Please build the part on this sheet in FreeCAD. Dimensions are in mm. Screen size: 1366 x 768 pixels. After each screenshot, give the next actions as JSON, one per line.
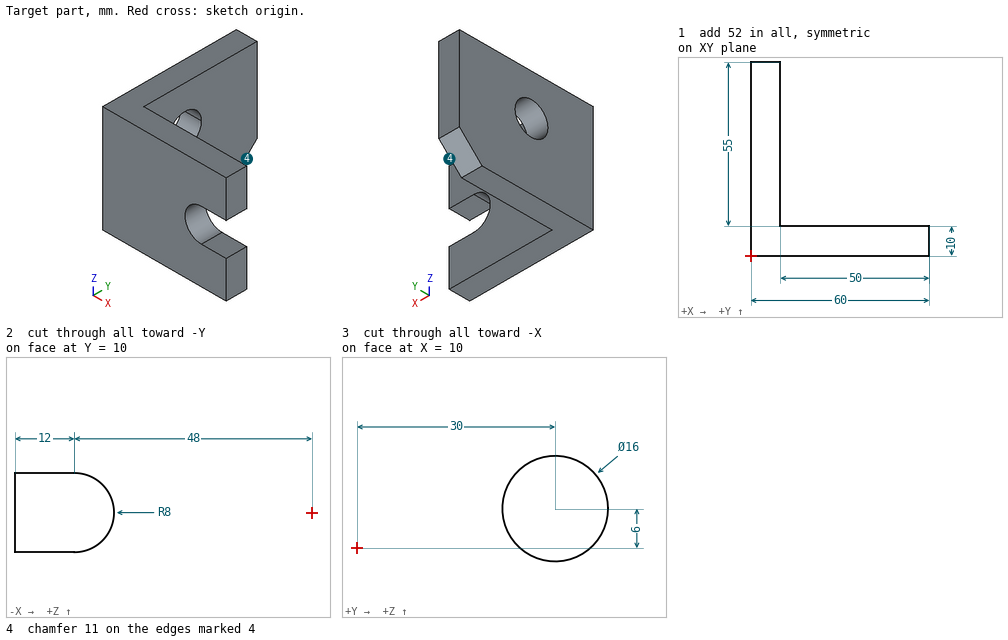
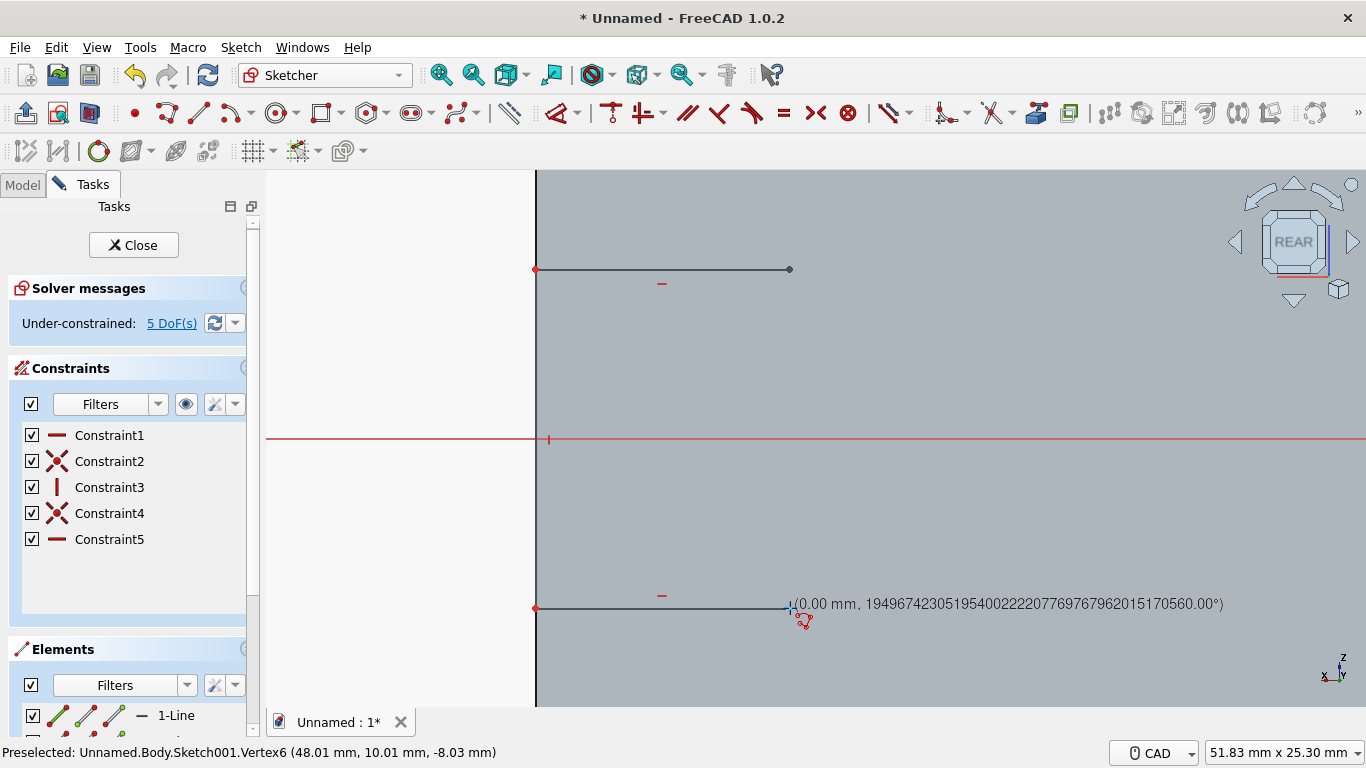
{"action": "key", "text": "g 3 a"}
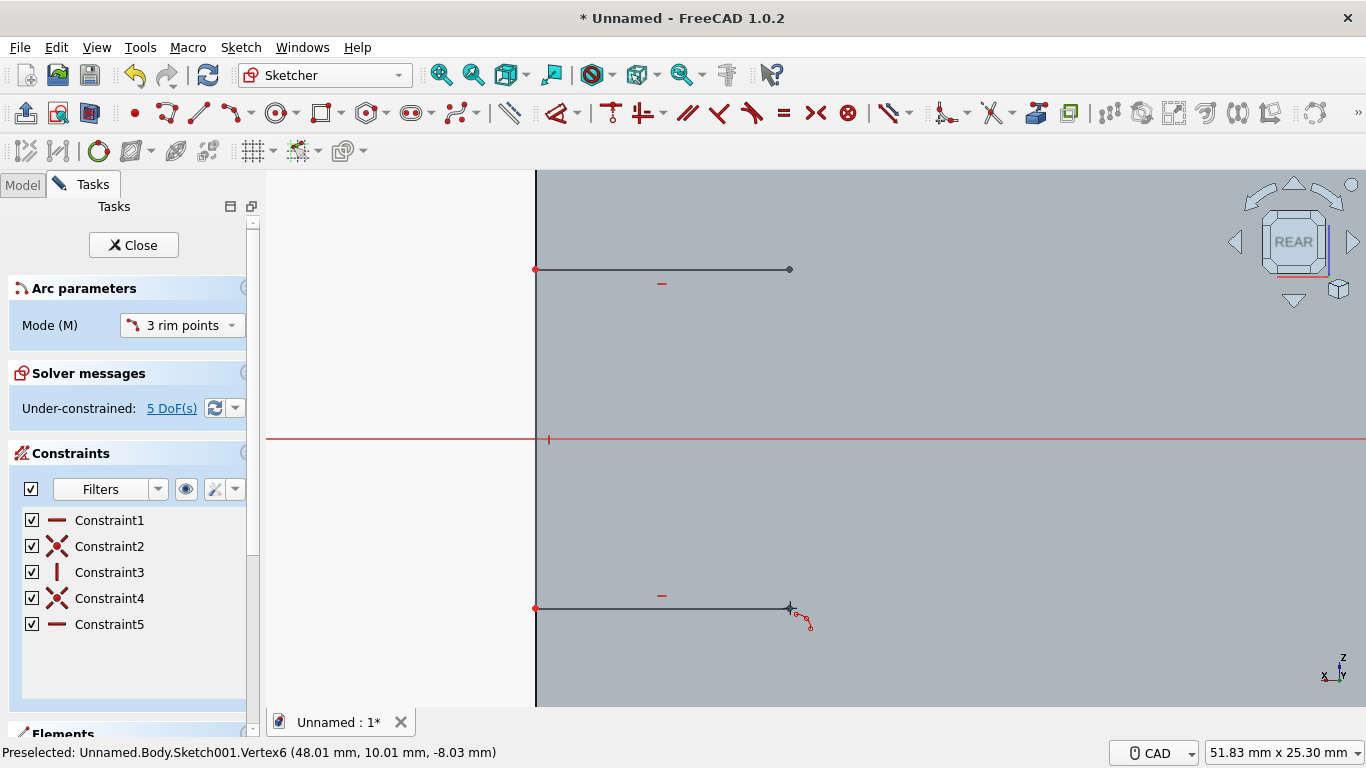
{"action": "left_click", "coordinate": [790, 609]}
{"action": "left_click", "coordinate": [790, 270]}
{"action": "left_click", "coordinate": [952, 491]}
{"action": "key", "text": "Escape"}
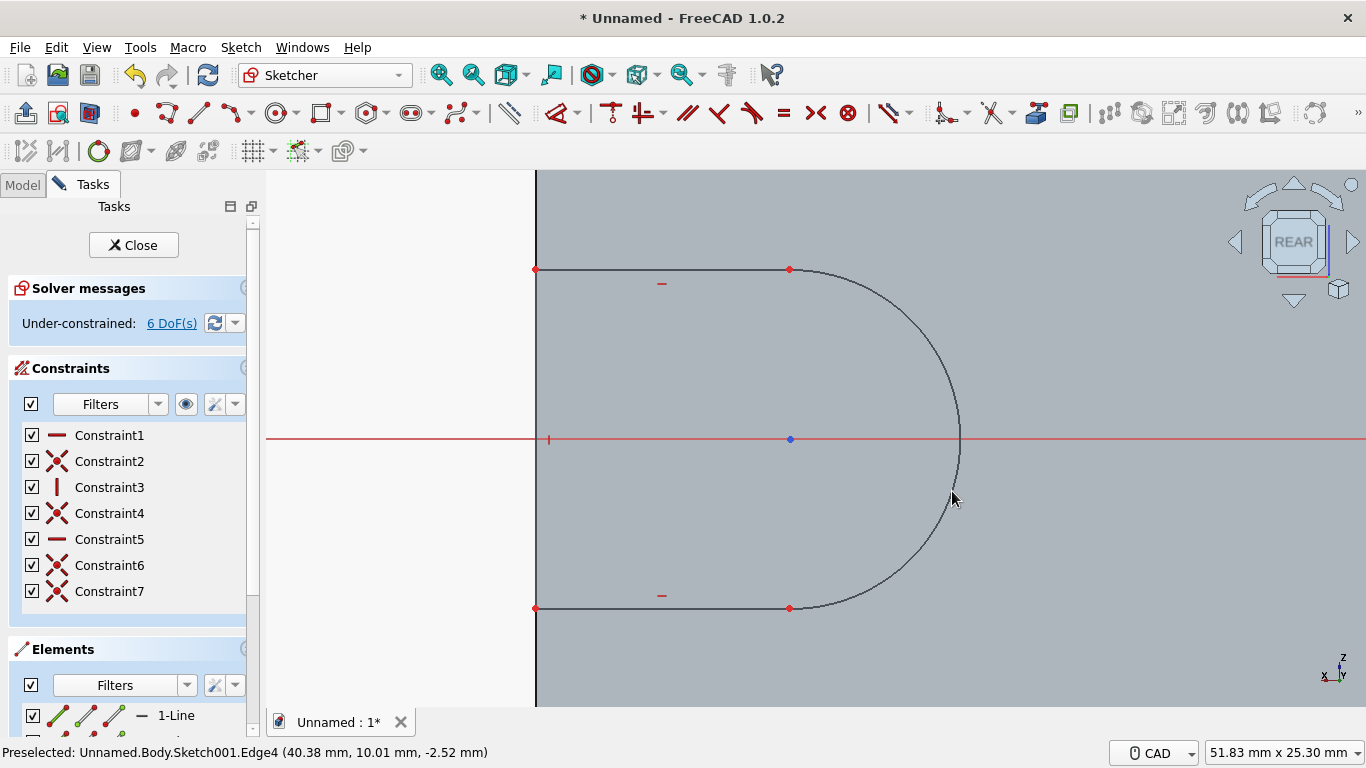
{"action": "left_click", "coordinate": [714, 270]}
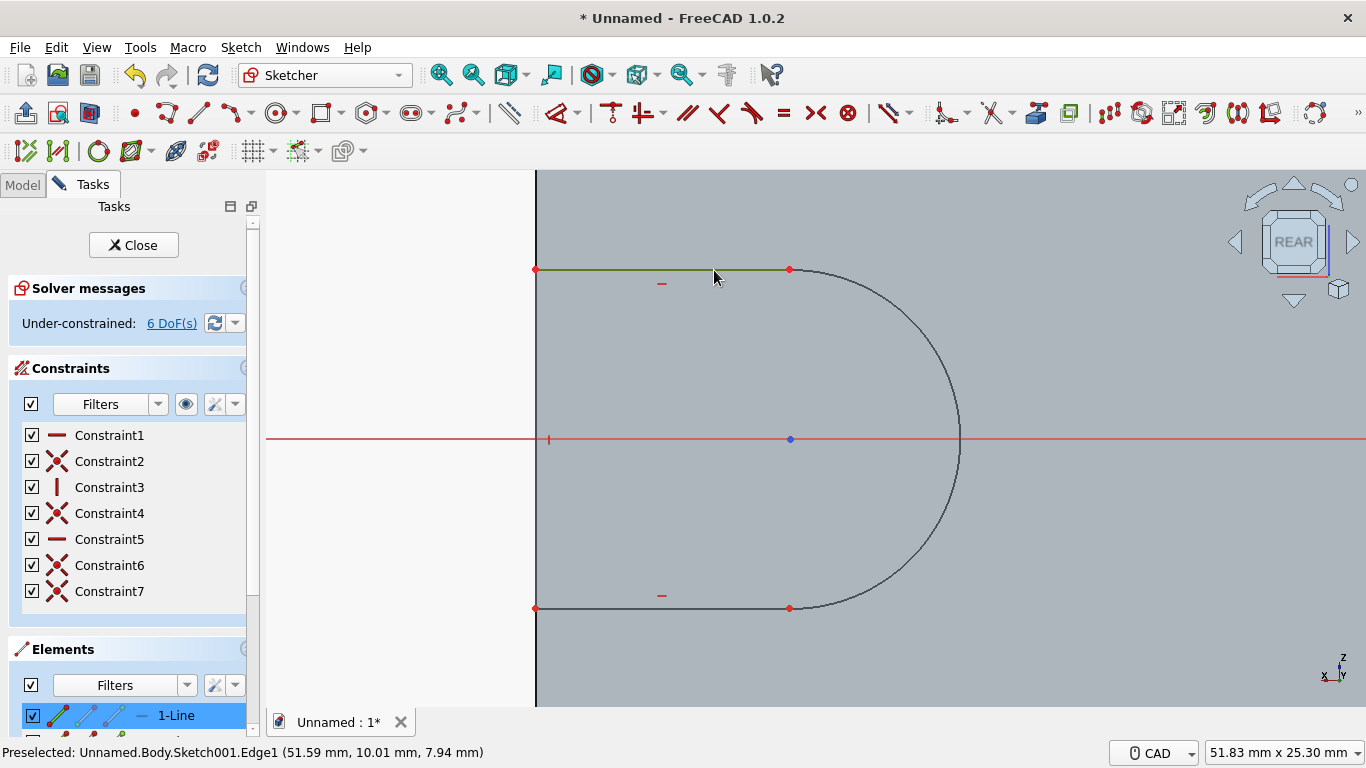
{"action": "left_click", "coordinate": [928, 539]}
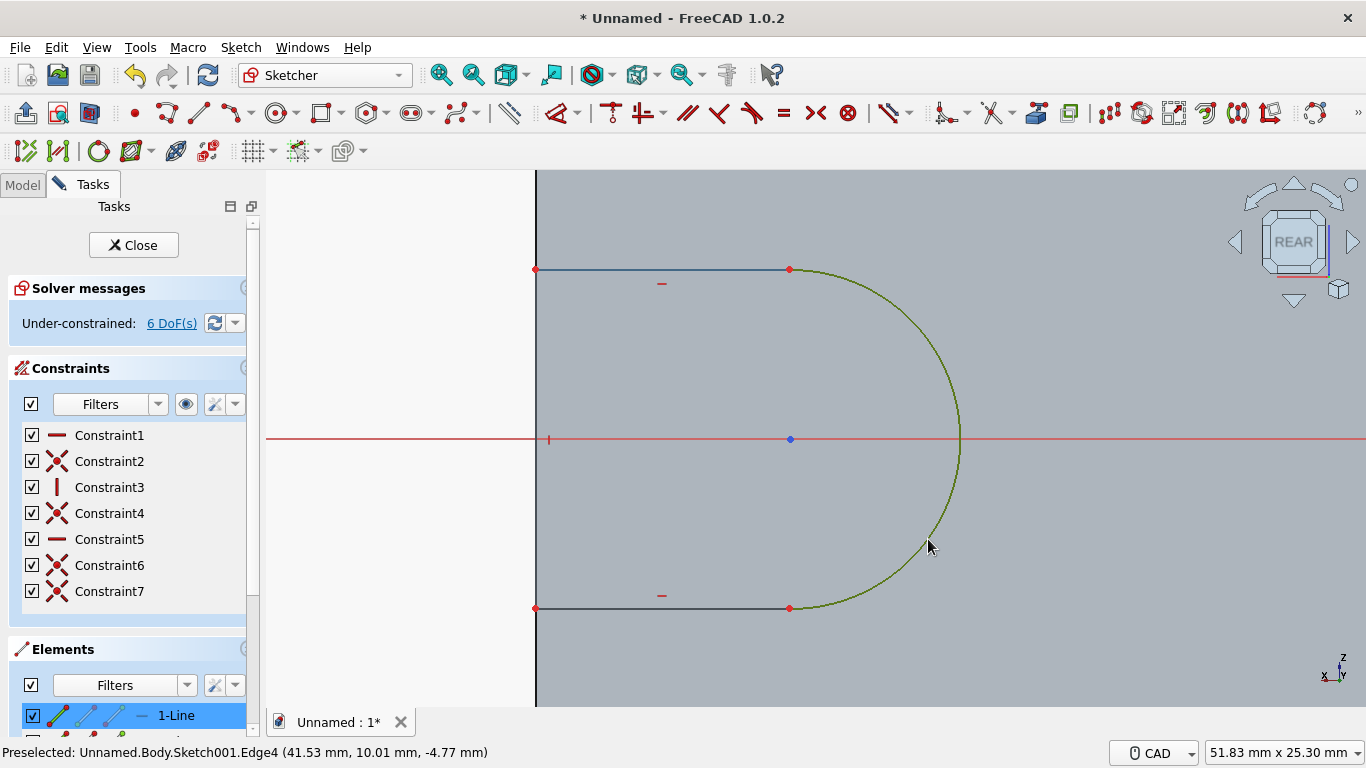
{"action": "left_click", "coordinate": [752, 114]}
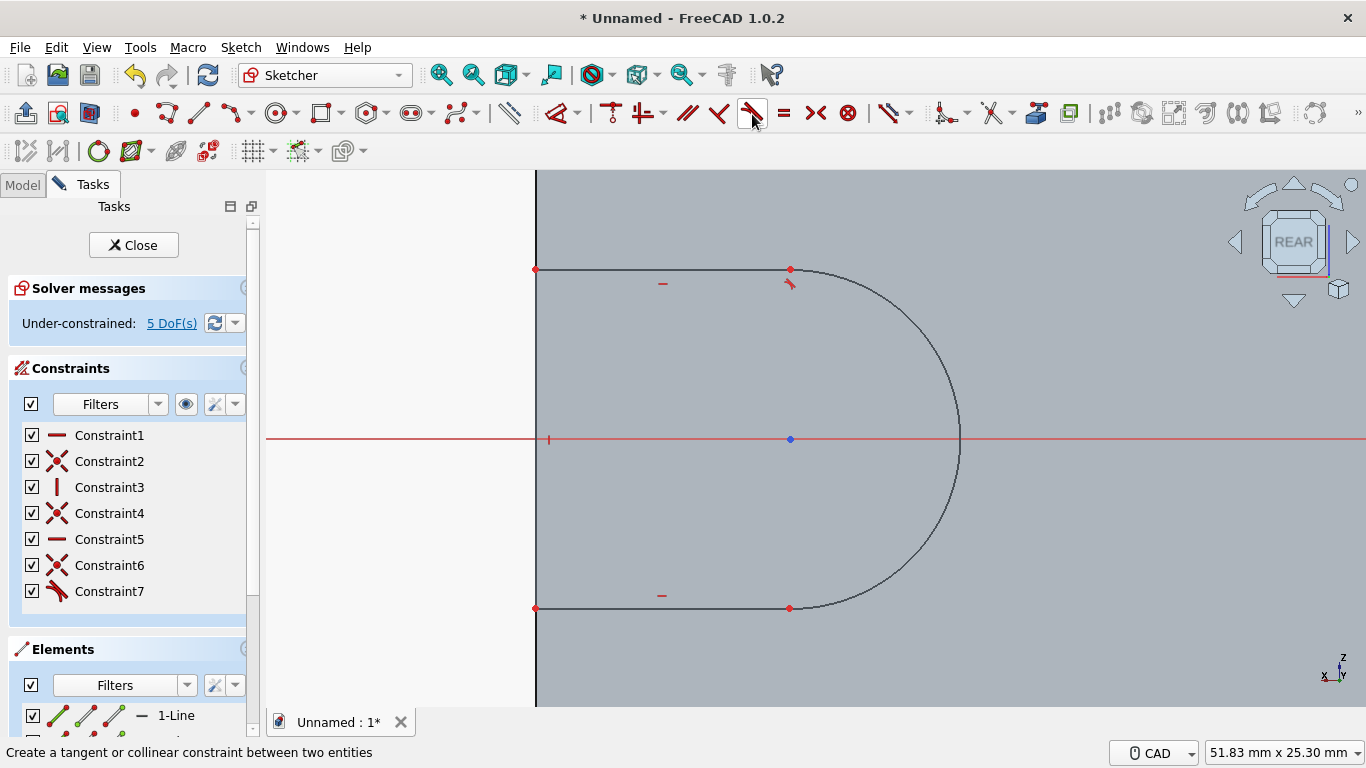
{"action": "left_click", "coordinate": [612, 609]}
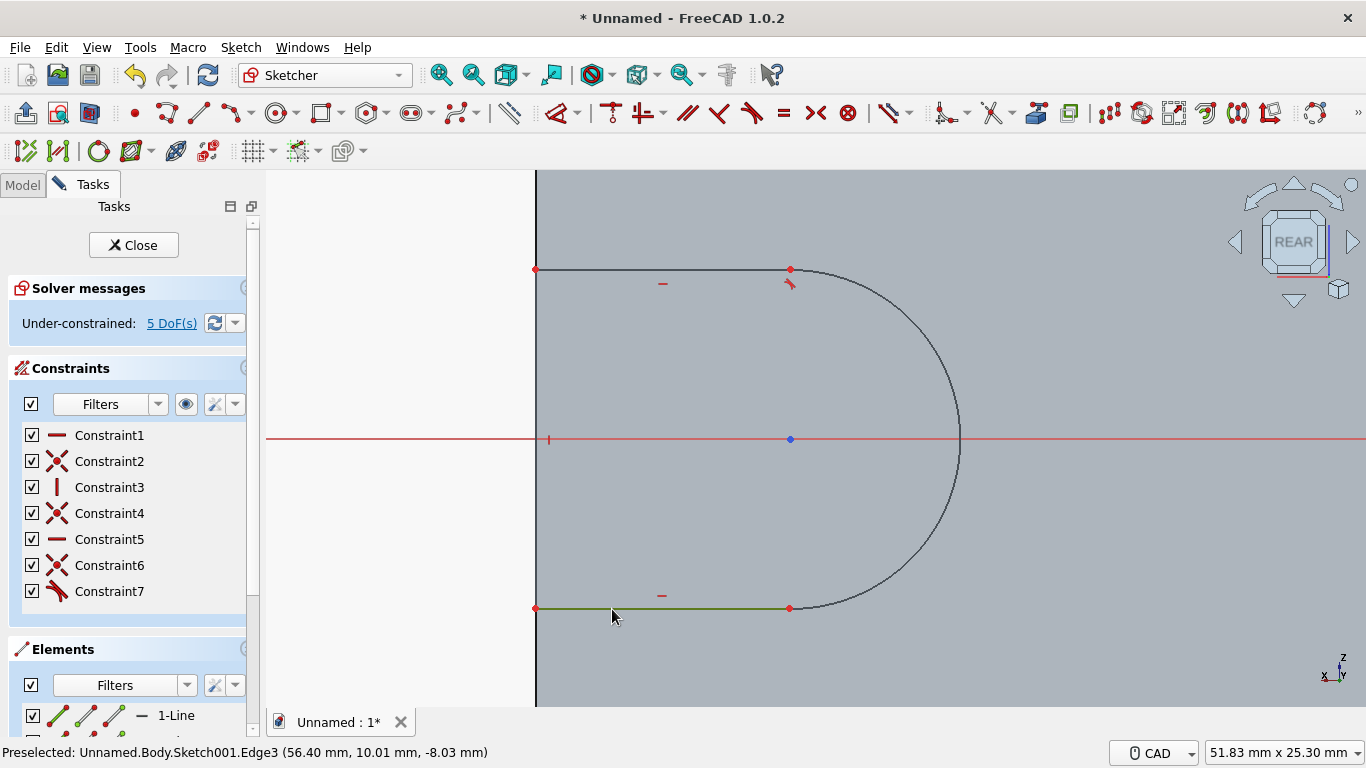
{"action": "left_click", "coordinate": [928, 540]}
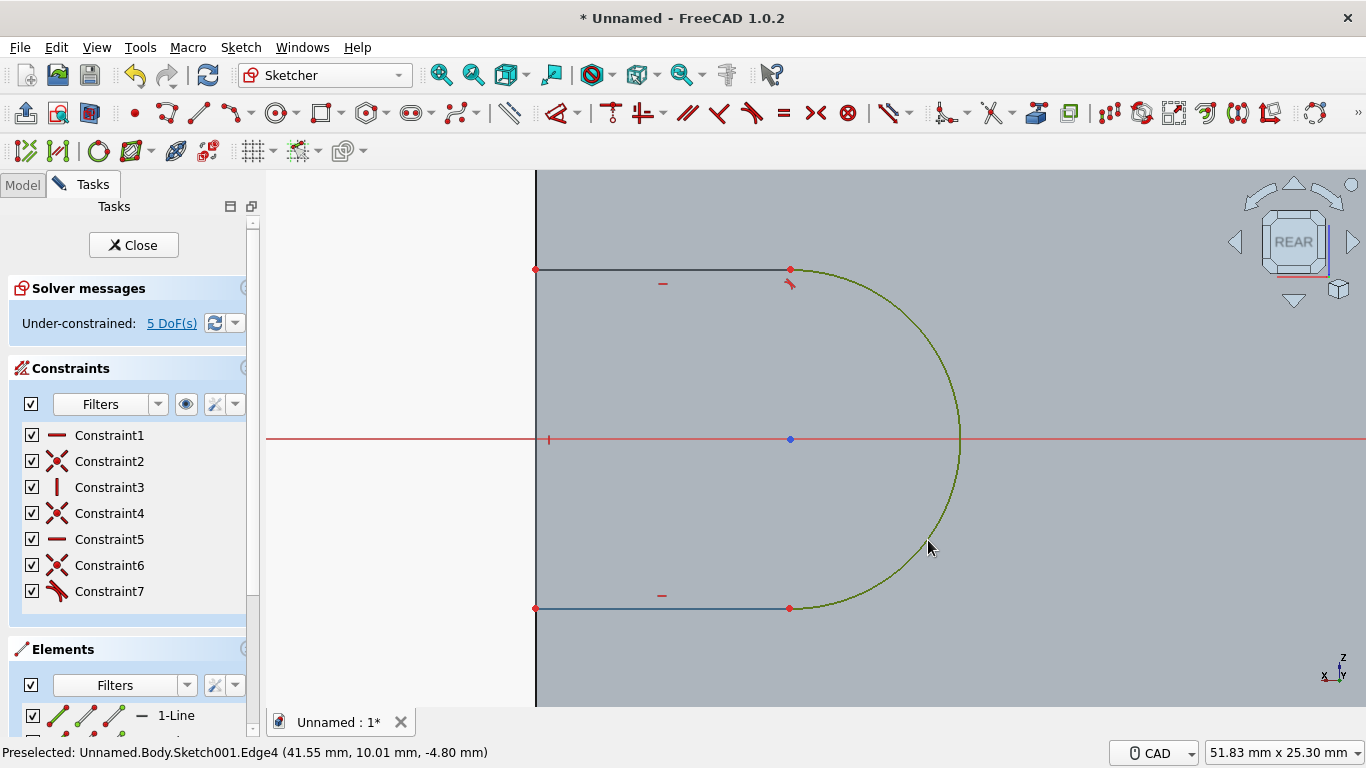
{"action": "left_click", "coordinate": [752, 114]}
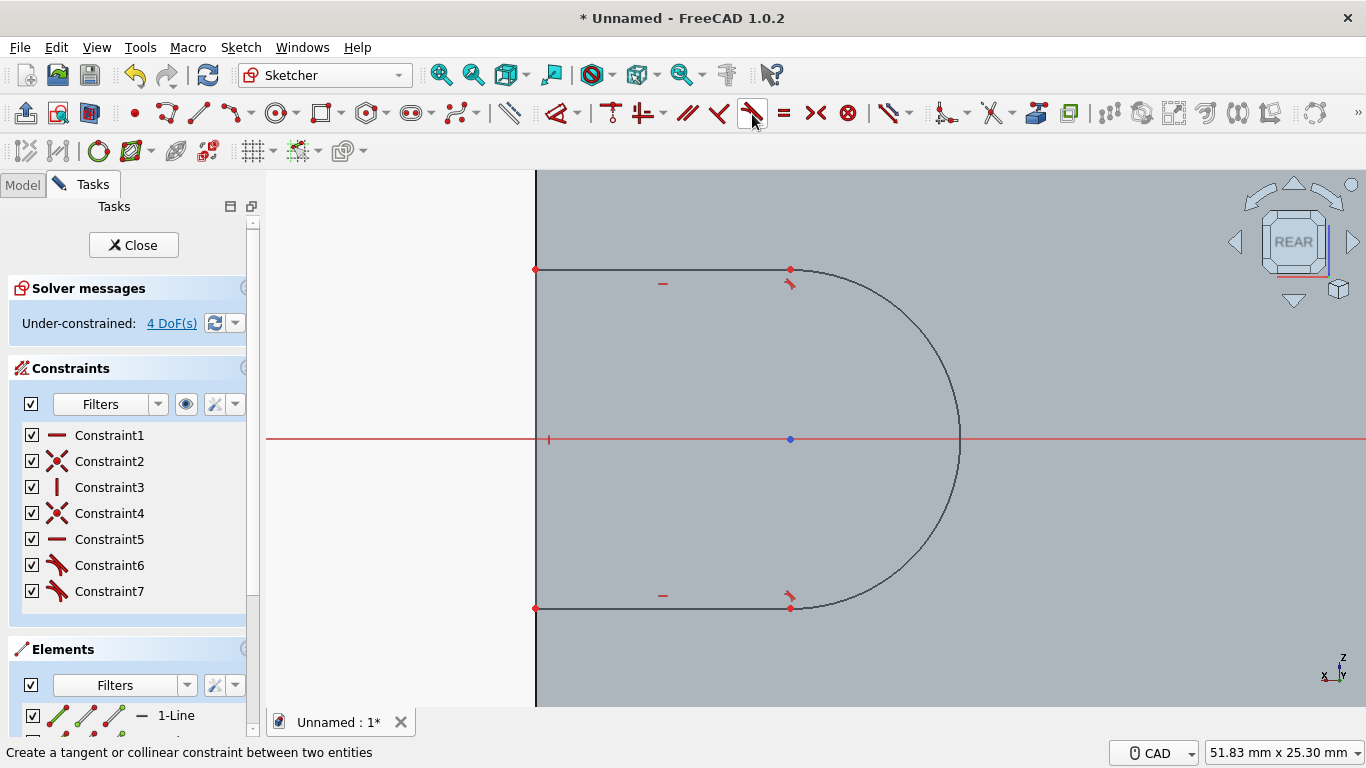
{"action": "left_click", "coordinate": [791, 439]}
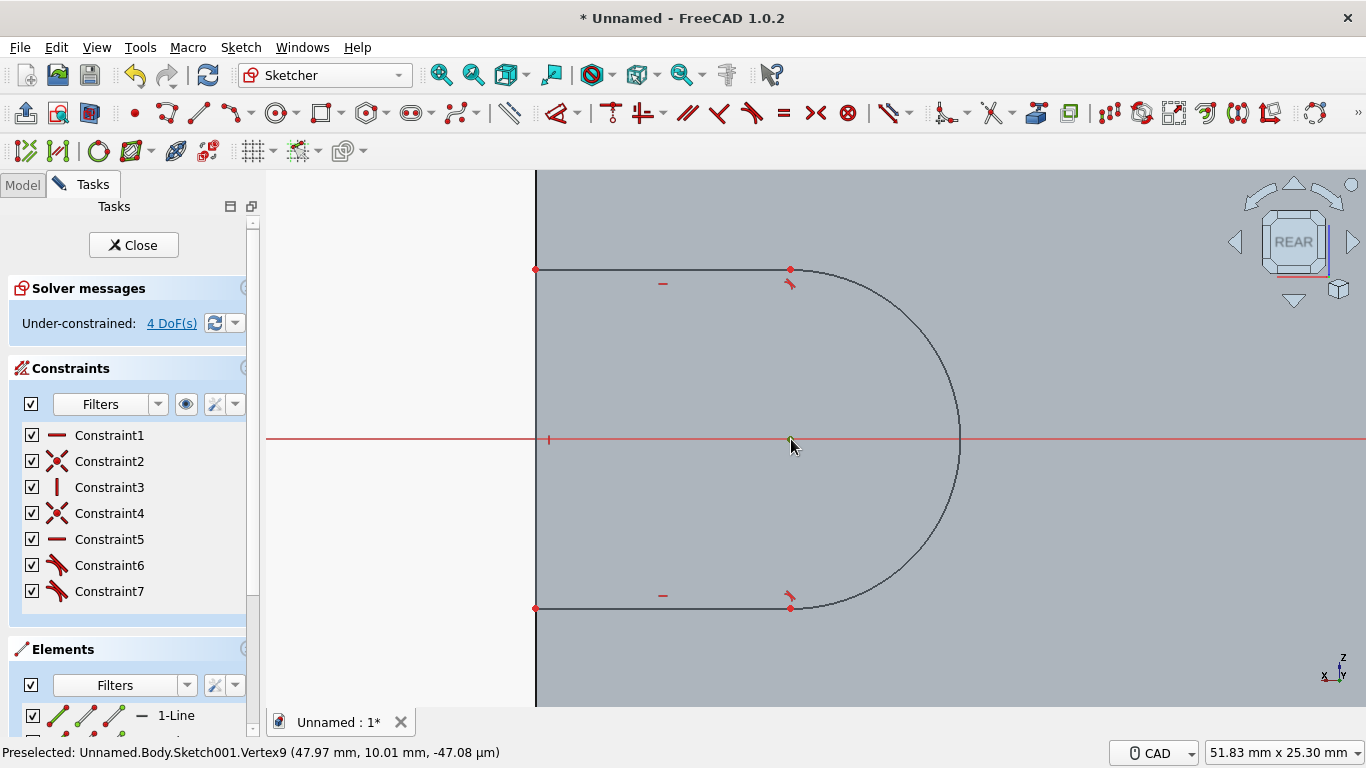
{"action": "left_click", "coordinate": [359, 438]}